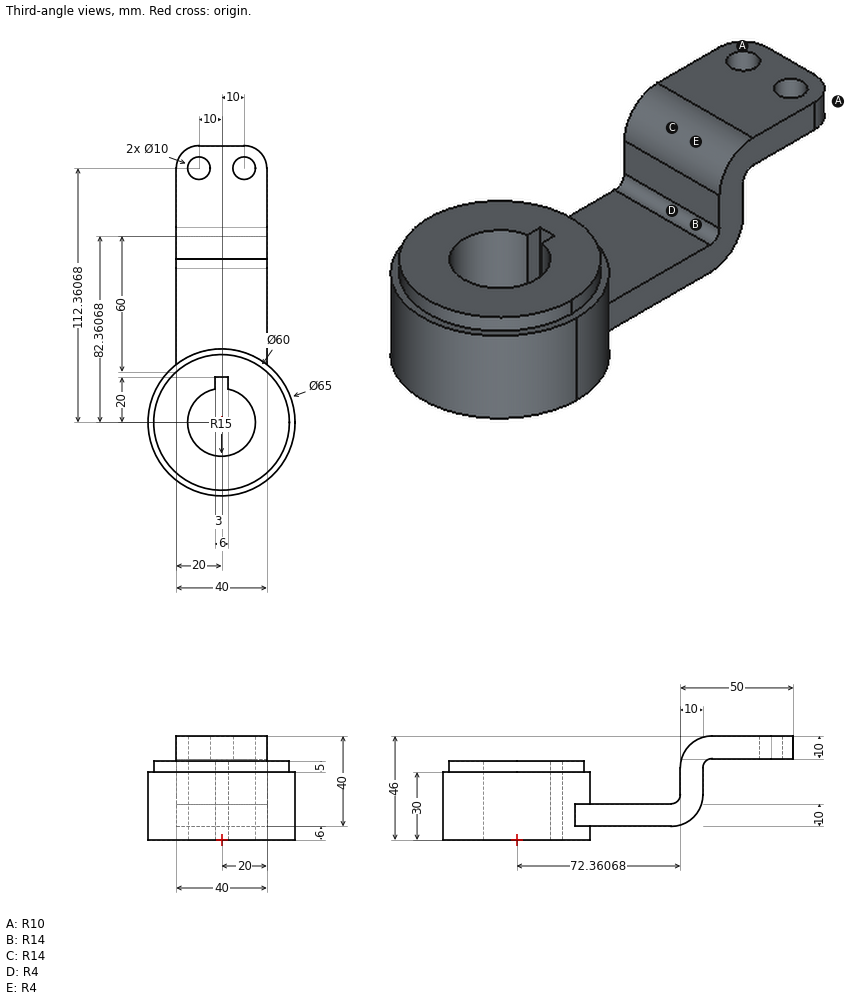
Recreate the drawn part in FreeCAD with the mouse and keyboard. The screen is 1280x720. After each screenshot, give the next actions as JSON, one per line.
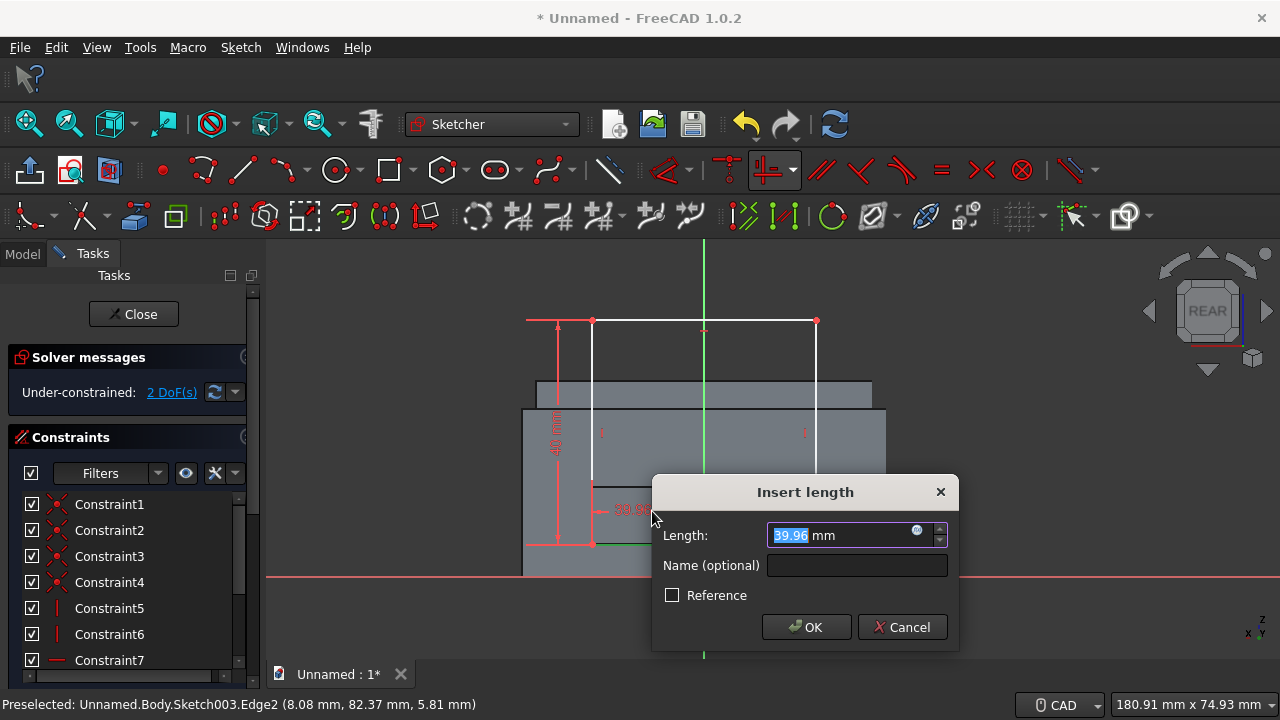
{"action": "type", "text": "40"}
{"action": "key", "text": "Return"}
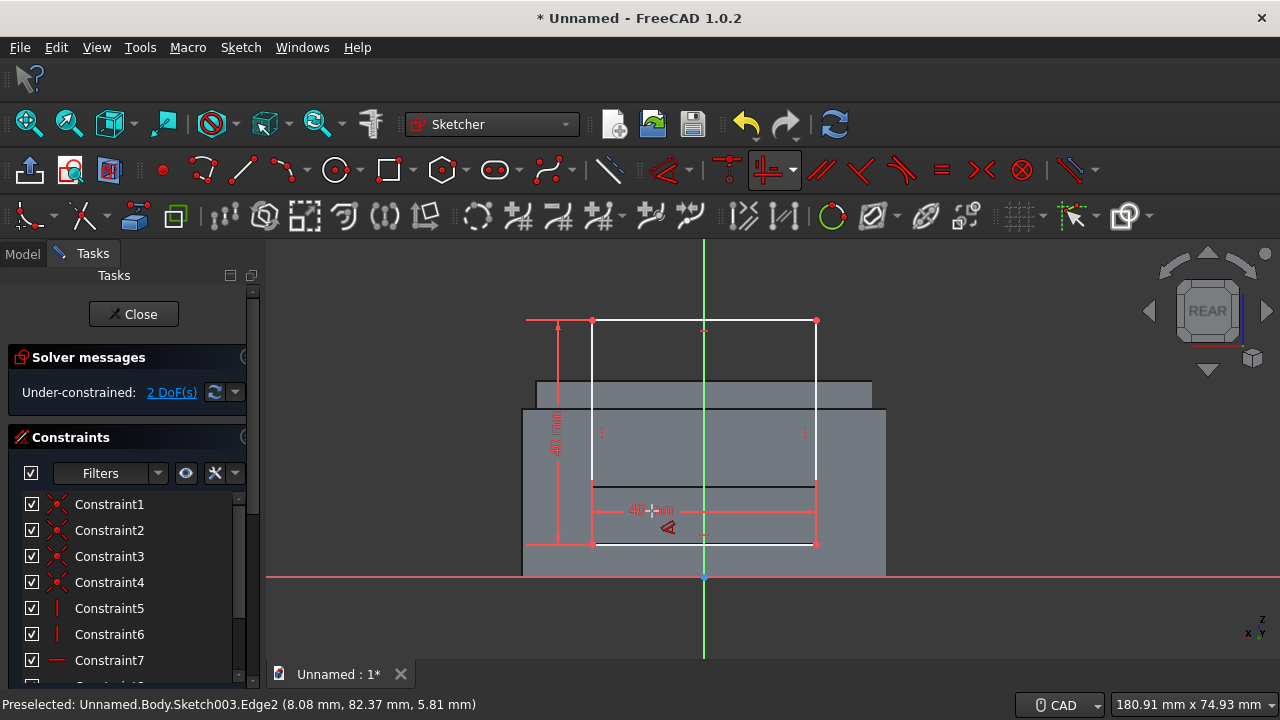
{"action": "left_click", "coordinate": [592, 545]}
{"action": "left_click", "coordinate": [558, 561]}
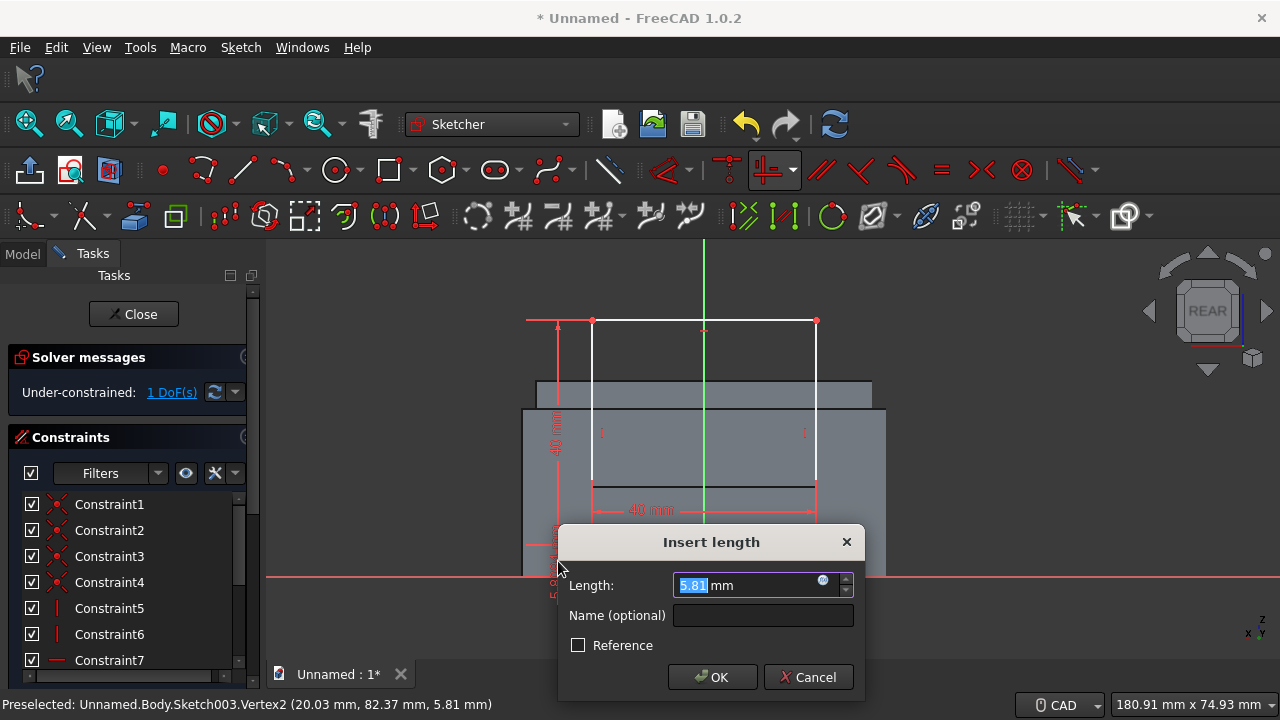
{"action": "type", "text": "6"}
{"action": "key", "text": "Return"}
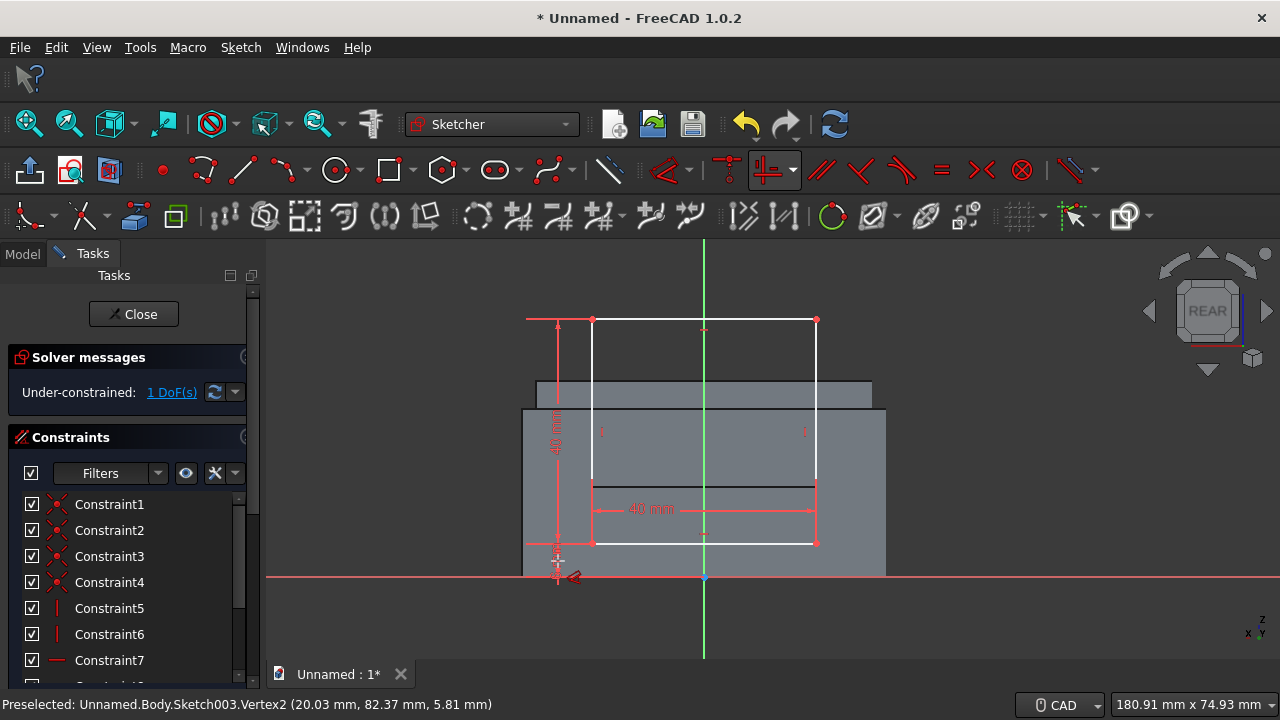
{"action": "left_click", "coordinate": [592, 319]}
{"action": "left_click", "coordinate": [648, 611]}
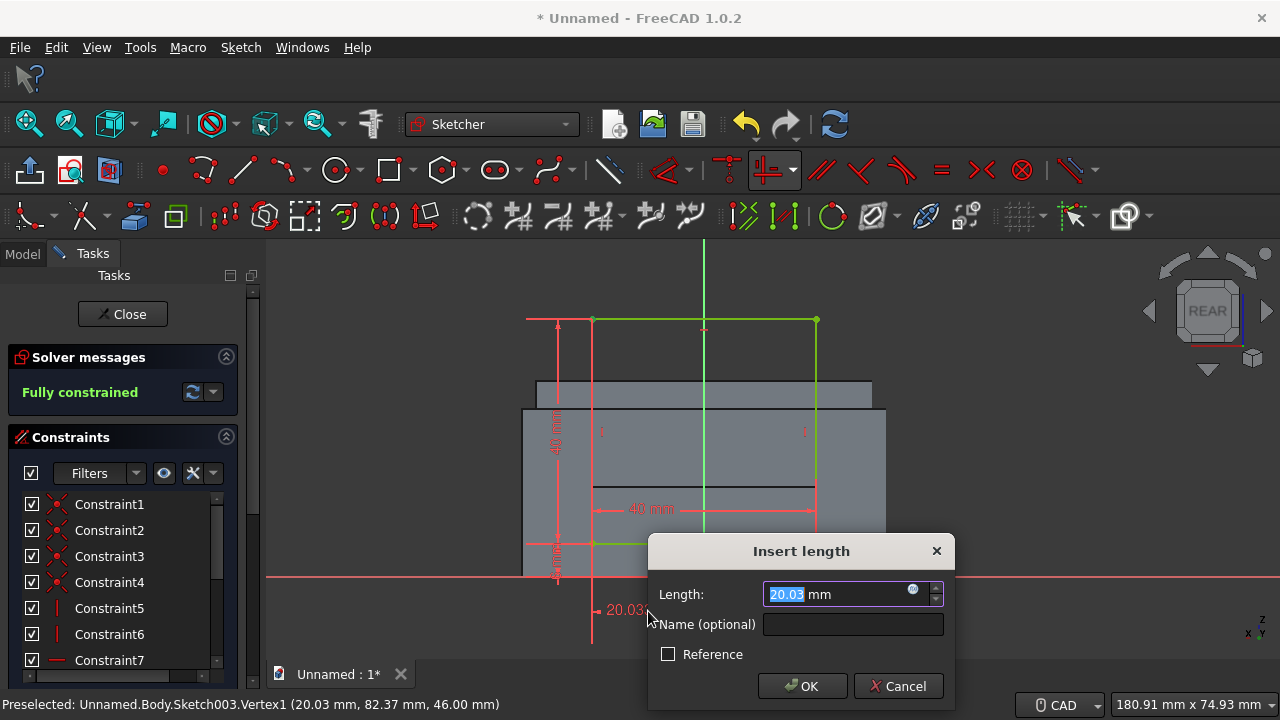
{"action": "type", "text": "20"}
{"action": "key", "text": "Return"}
{"action": "key", "text": "Escape"}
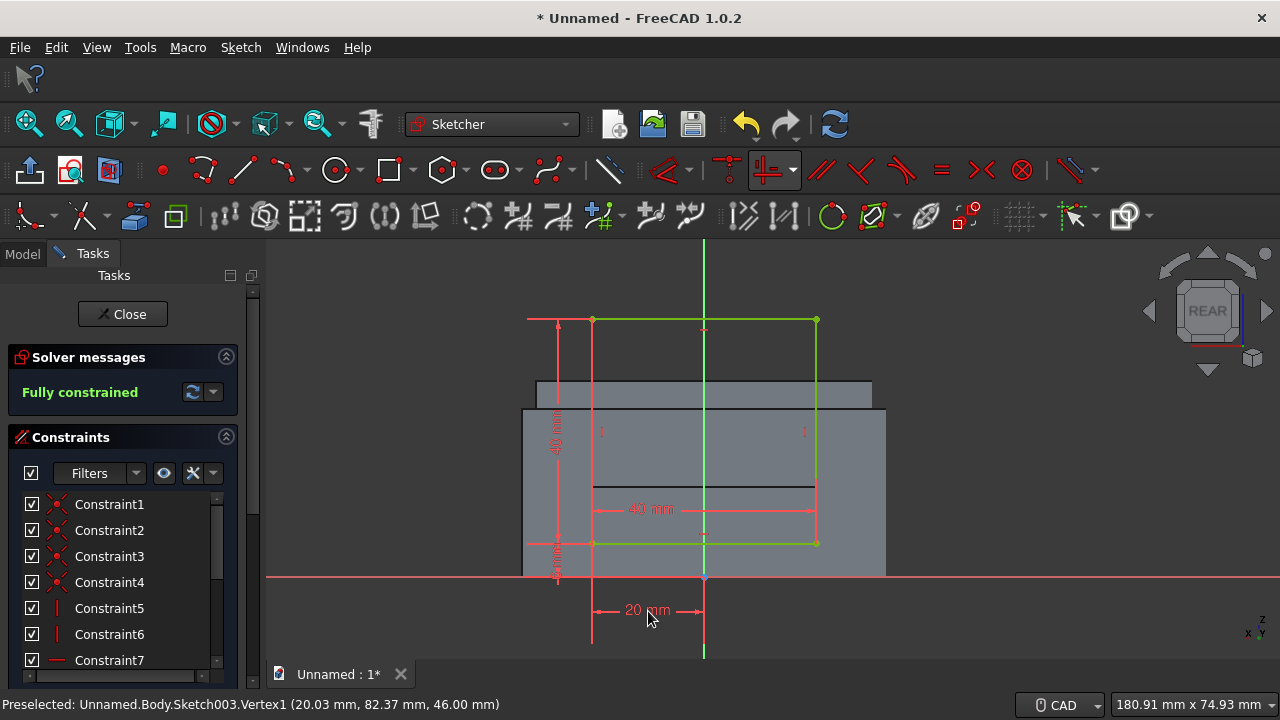
{"action": "left_click", "coordinate": [123, 314]}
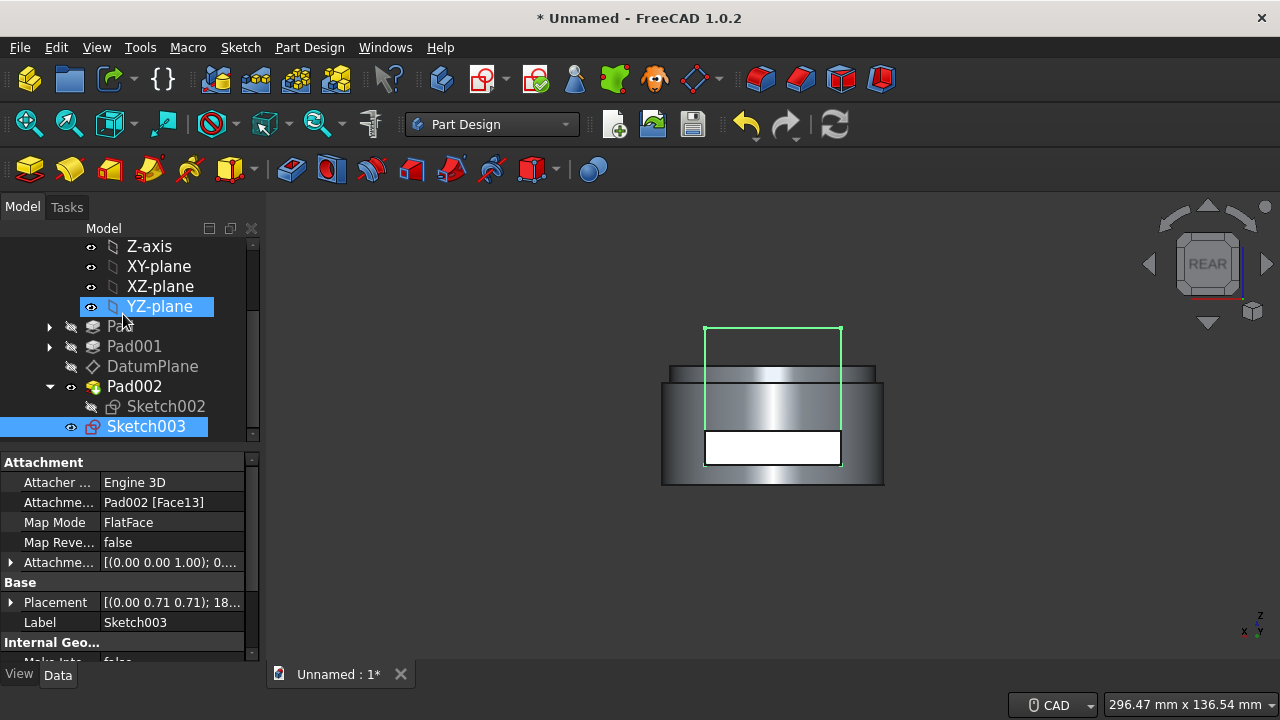
{"action": "left_click", "coordinate": [30, 170]}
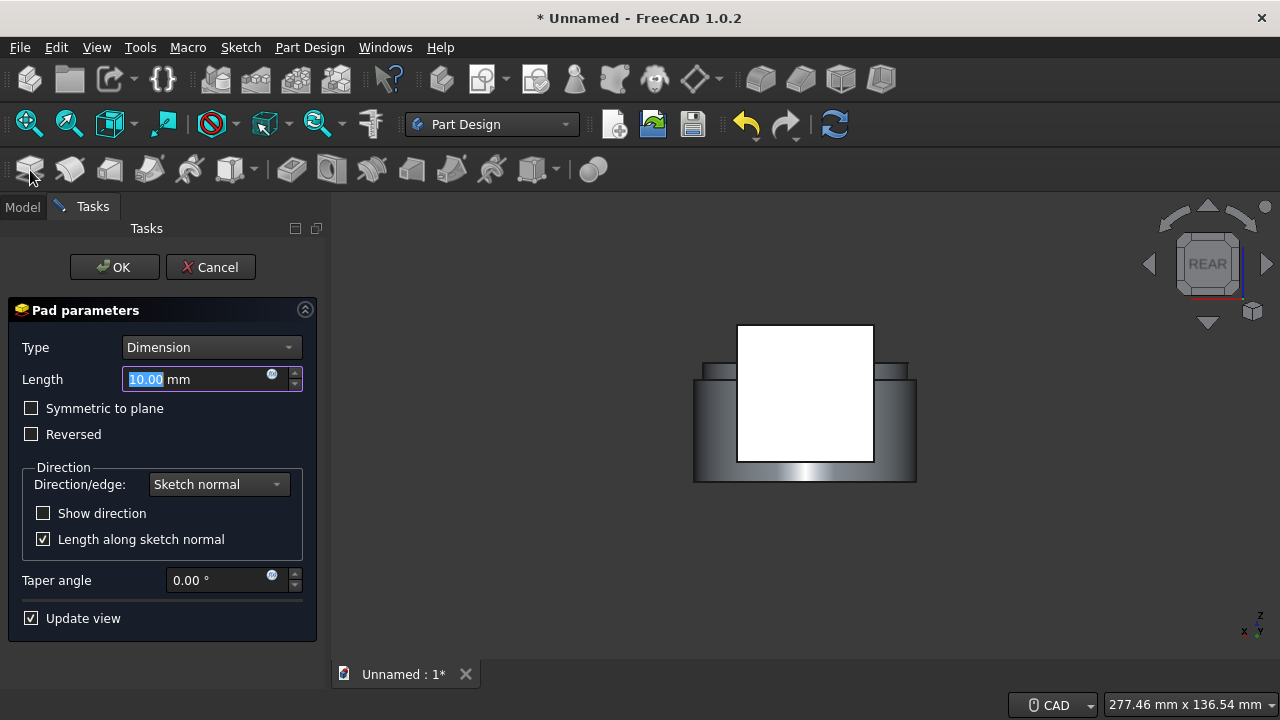
{"action": "type", "text": "10"}
{"action": "key", "text": "Tab"}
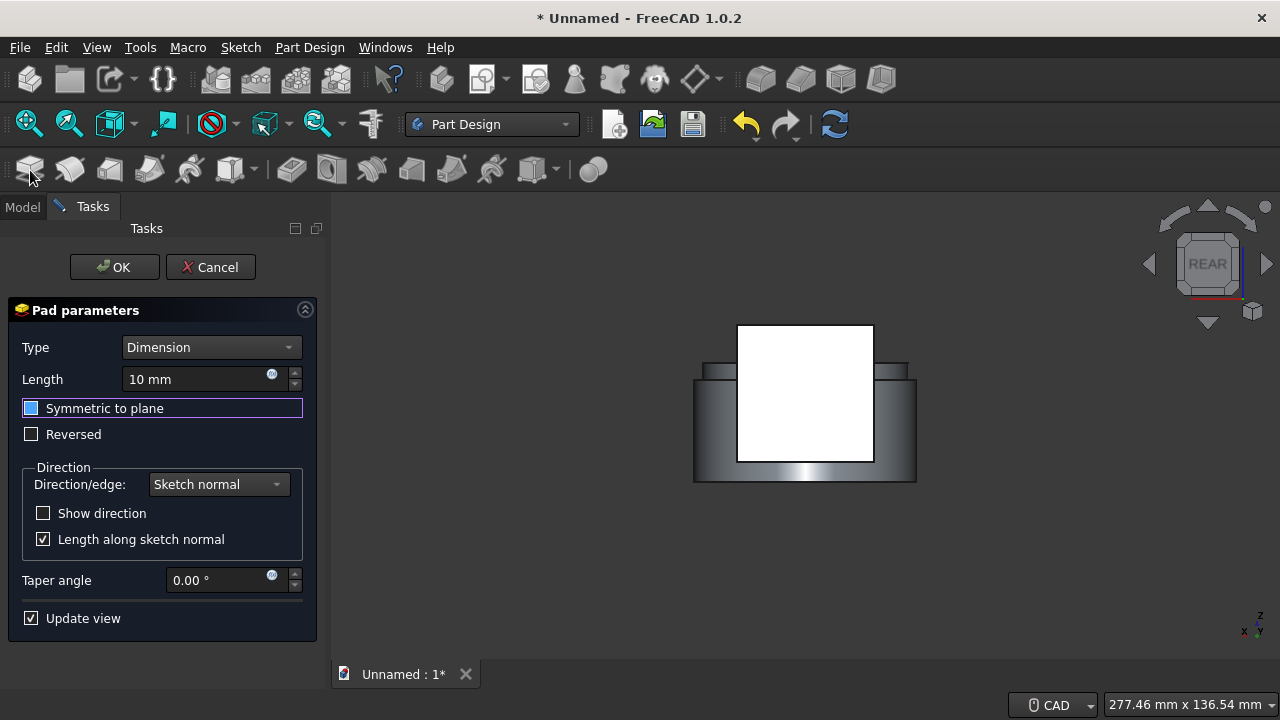
{"action": "left_click", "coordinate": [30, 434]}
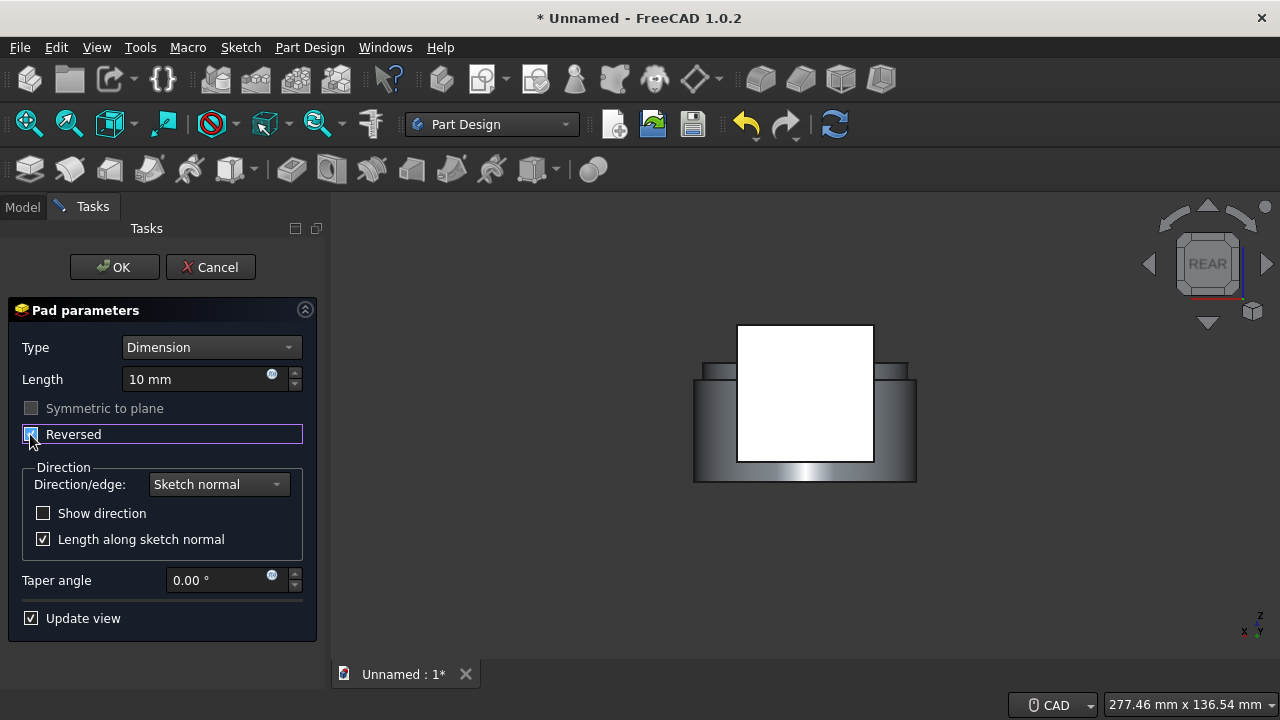
{"action": "left_click", "coordinate": [115, 267]}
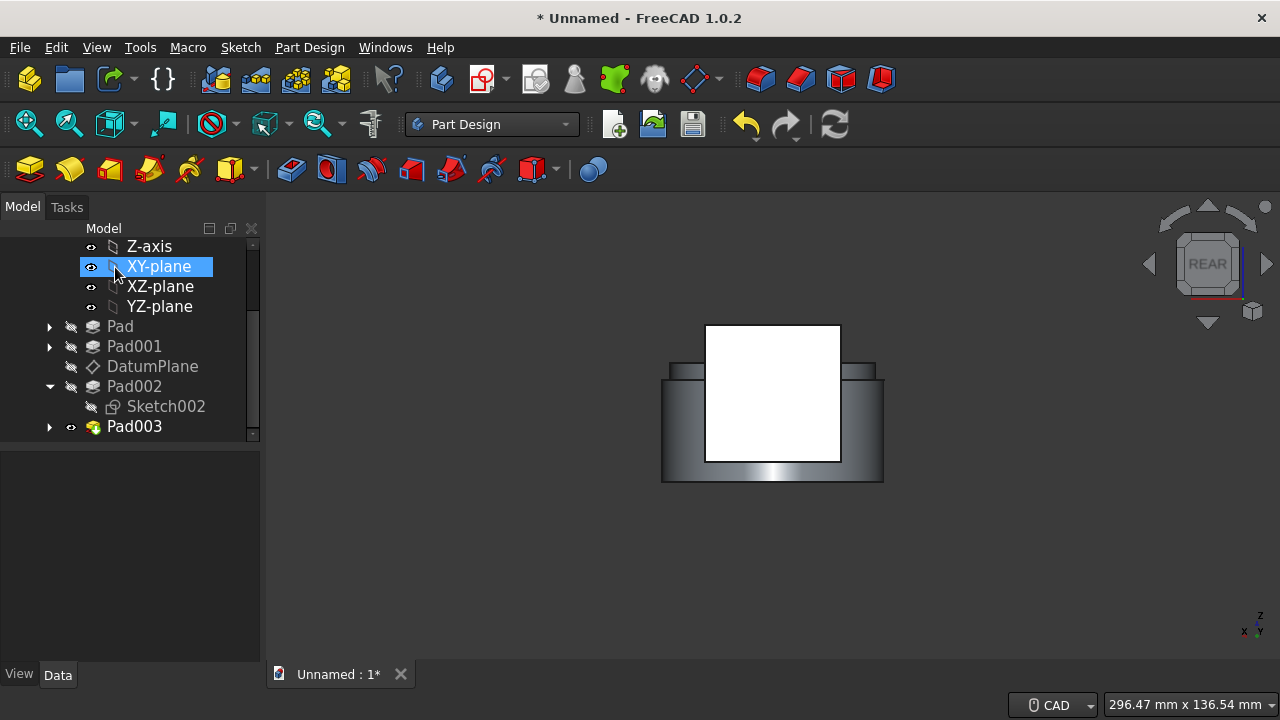
{"action": "key", "text": "v f"}